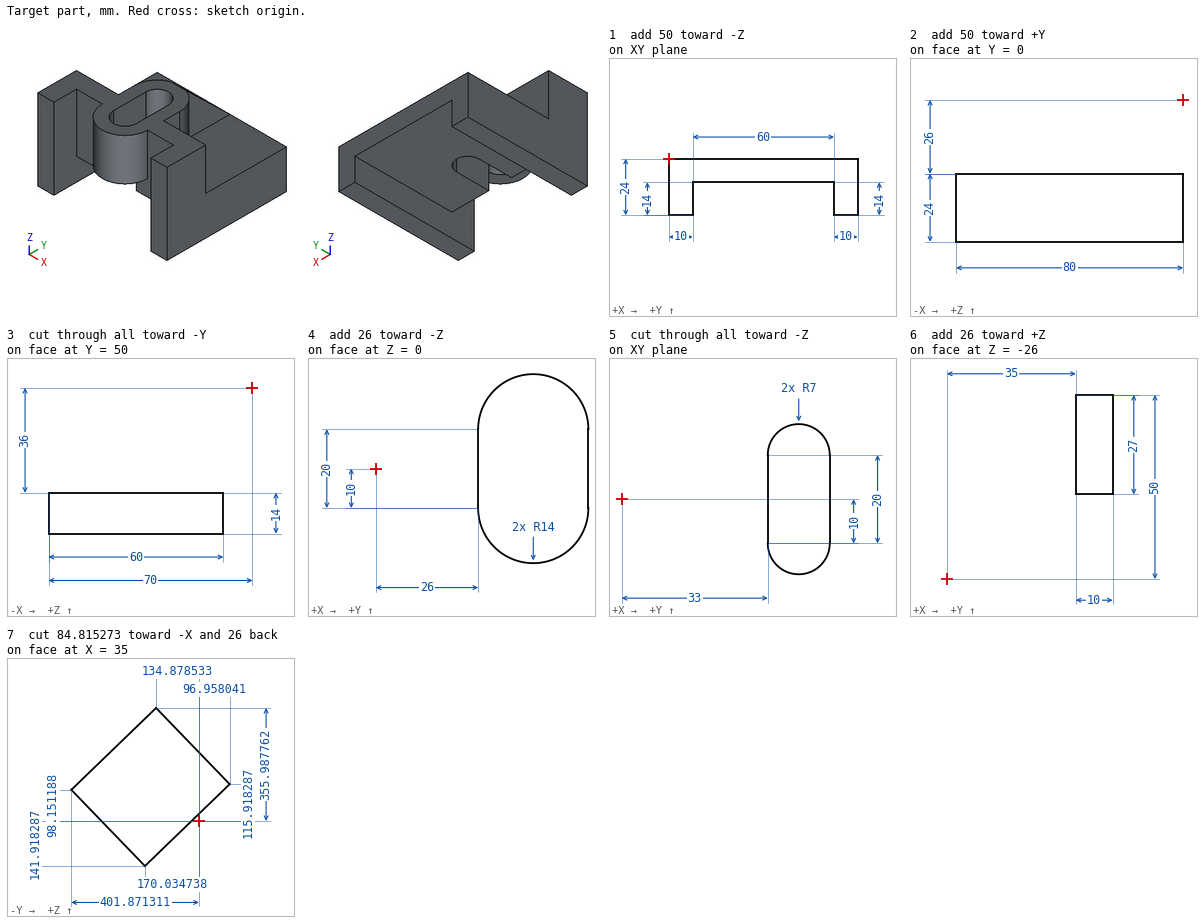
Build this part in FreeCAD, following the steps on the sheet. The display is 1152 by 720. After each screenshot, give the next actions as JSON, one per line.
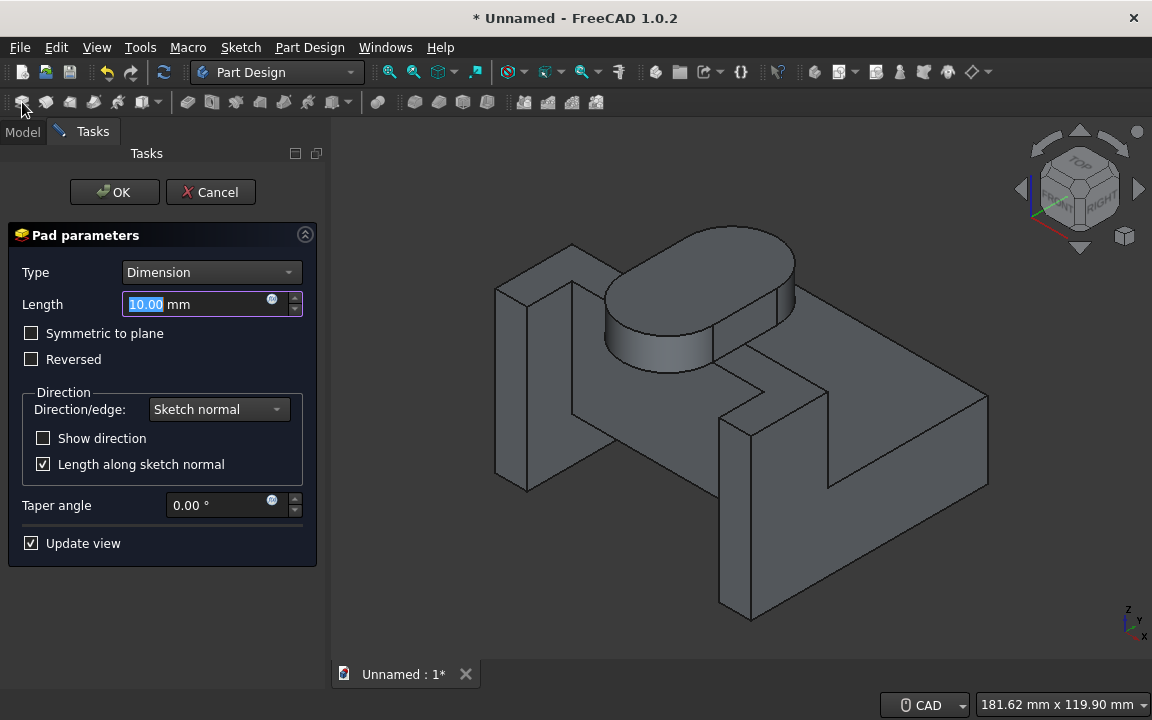
{"action": "type", "text": "26"}
{"action": "key", "text": "Tab"}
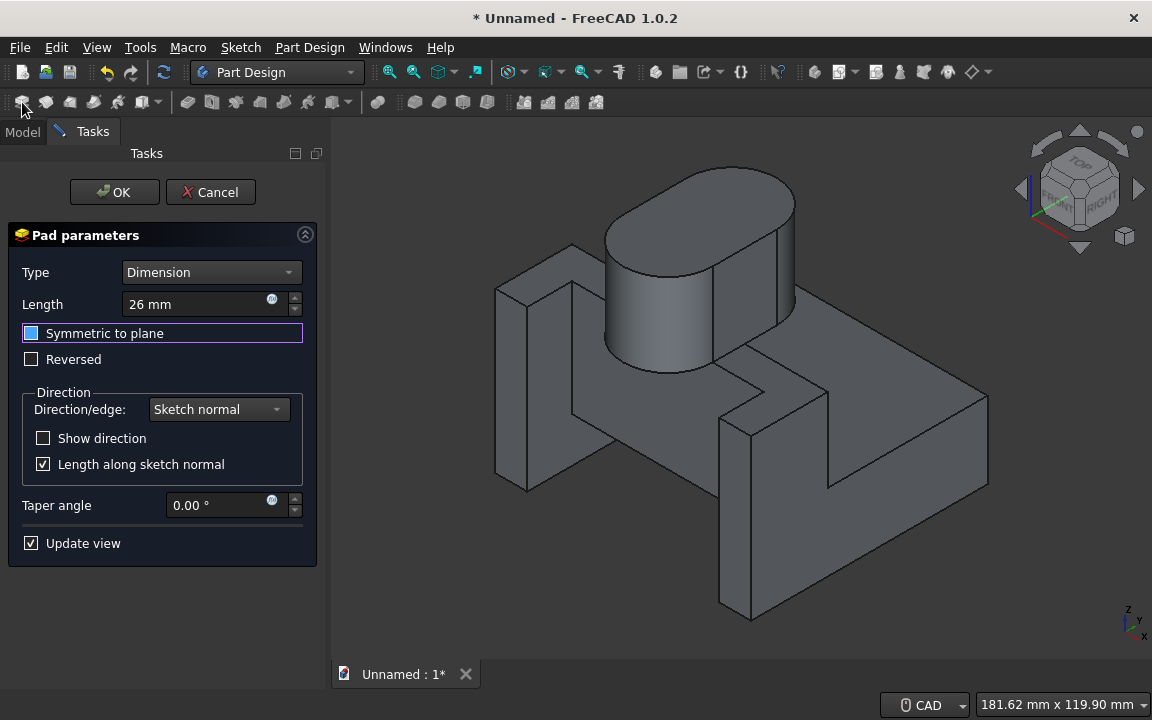
{"action": "left_click", "coordinate": [30, 359]}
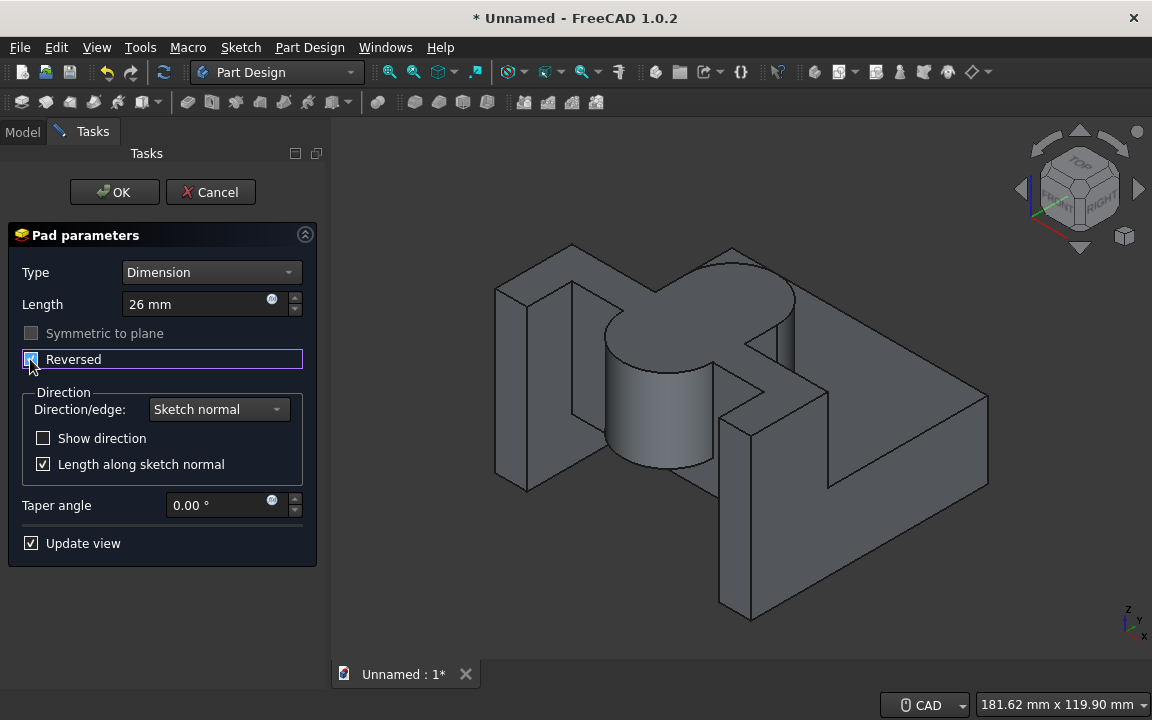
{"action": "left_click", "coordinate": [115, 192]}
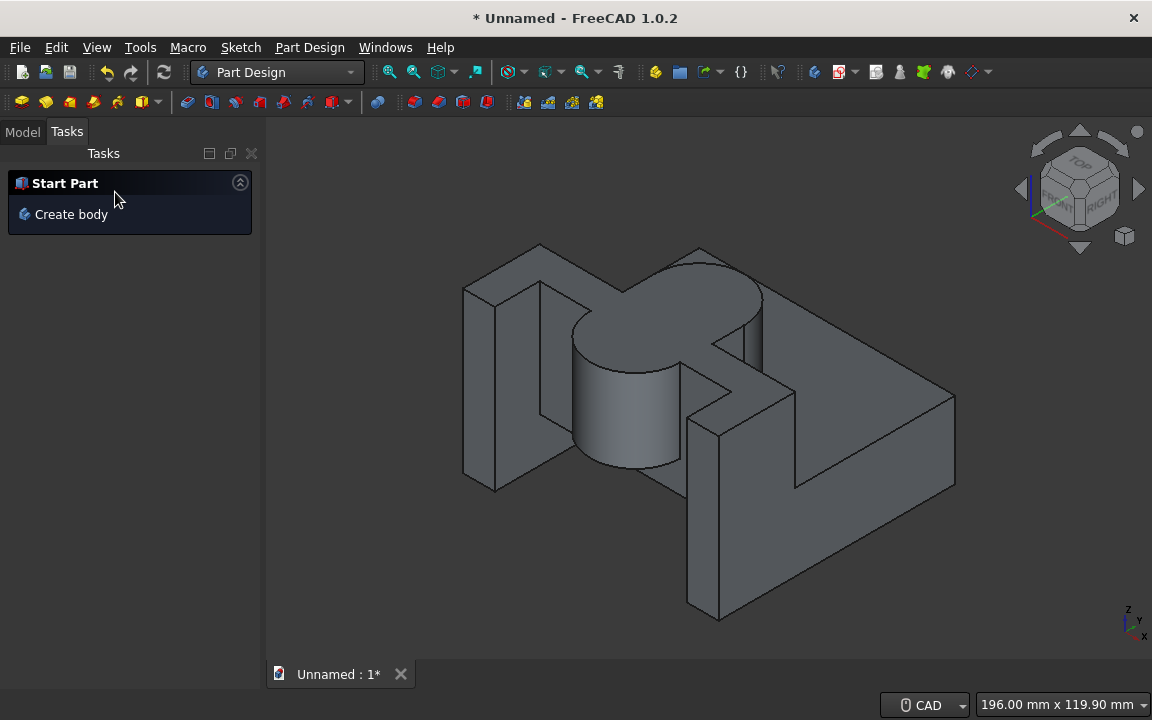
{"action": "left_click", "coordinate": [840, 72]}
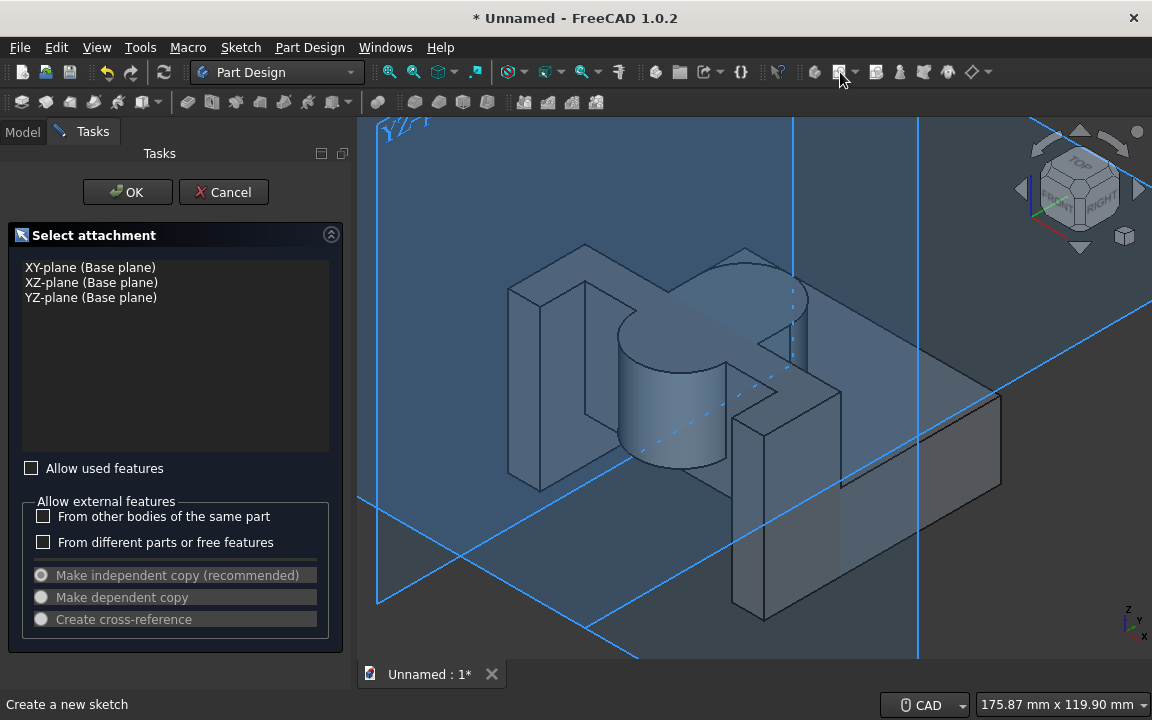
{"action": "left_click", "coordinate": [82, 268]}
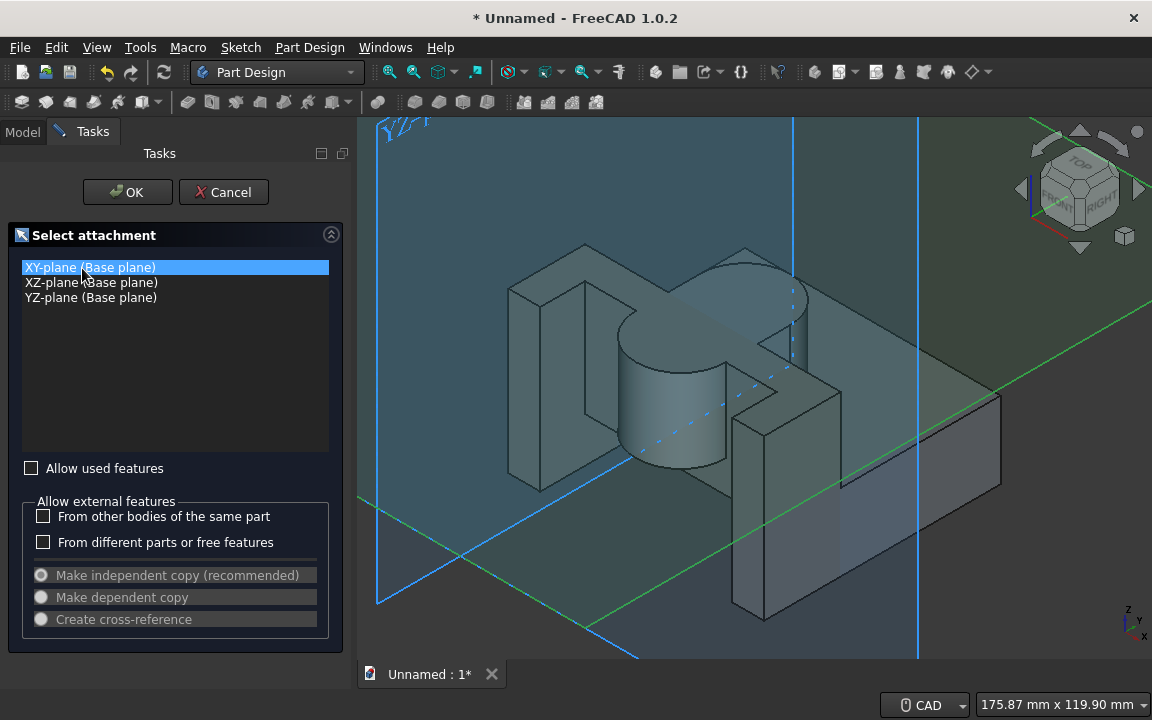
{"action": "left_click", "coordinate": [128, 192]}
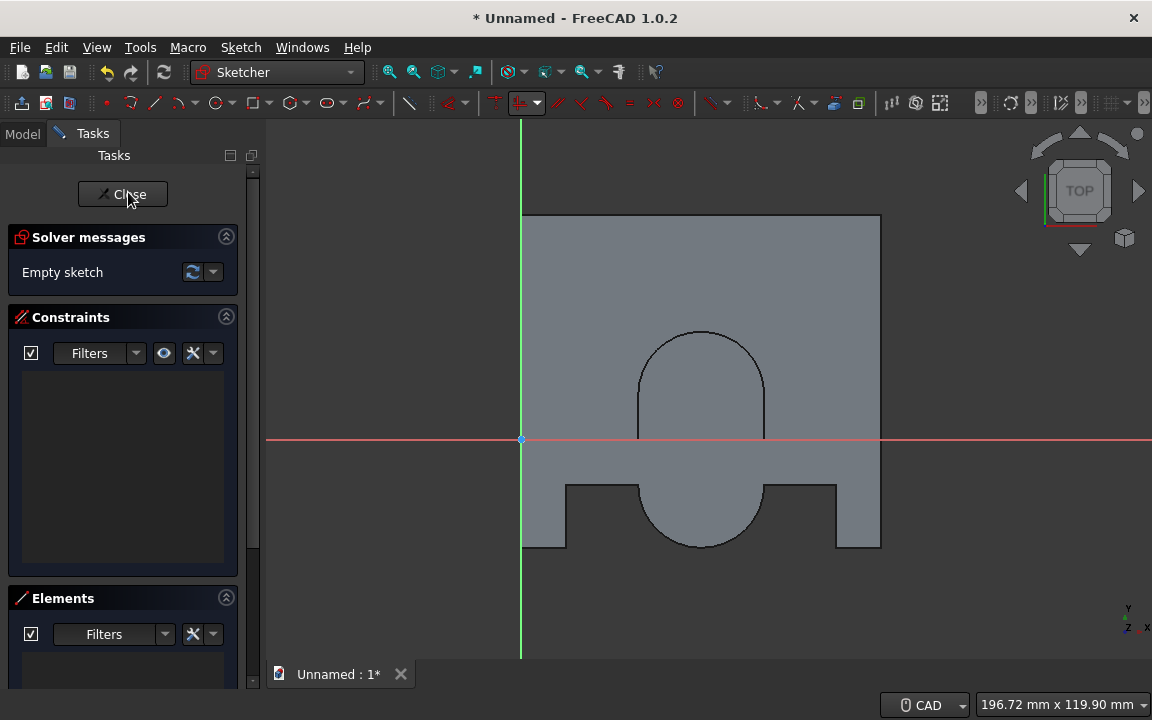
{"action": "scroll", "coordinate": [616, 481], "scroll_direction": "up", "scroll_amount": 4}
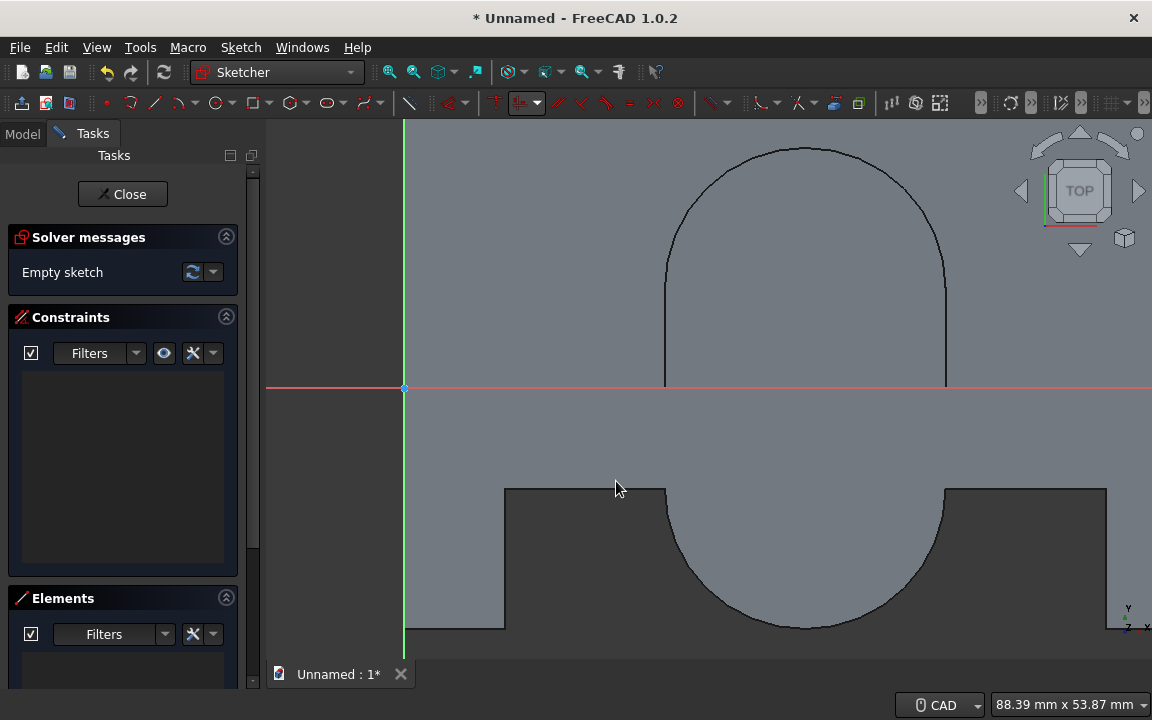
{"action": "key", "text": "g s"}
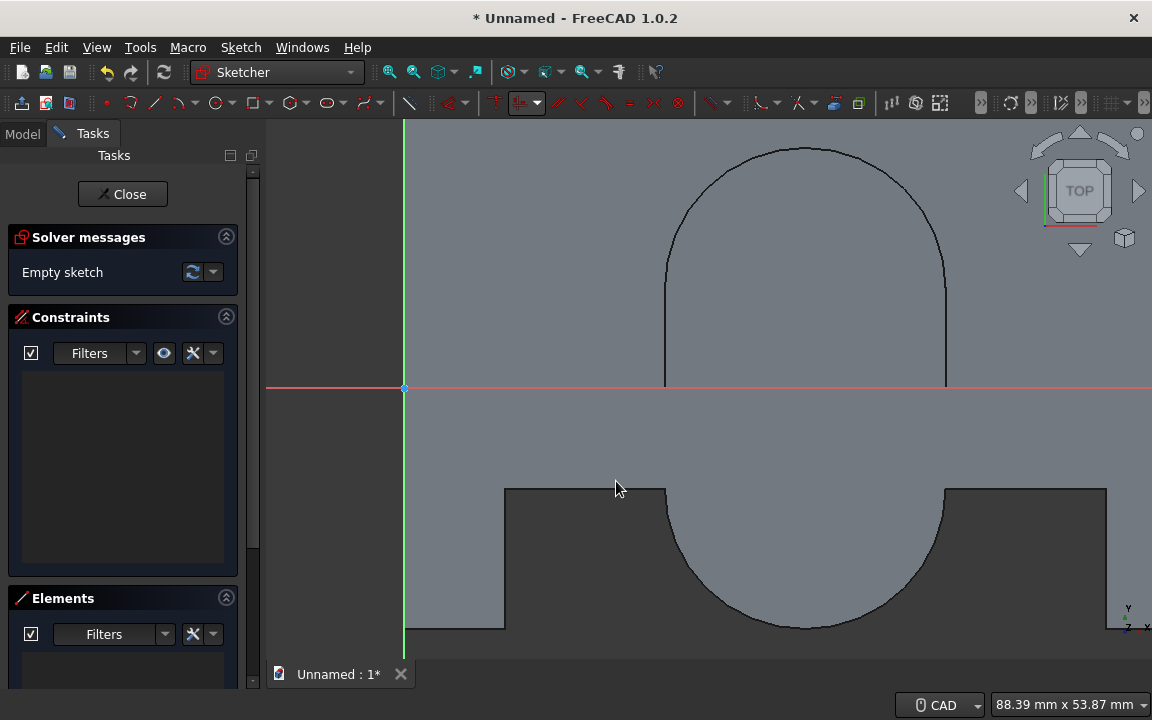
{"action": "left_click", "coordinate": [805, 489]}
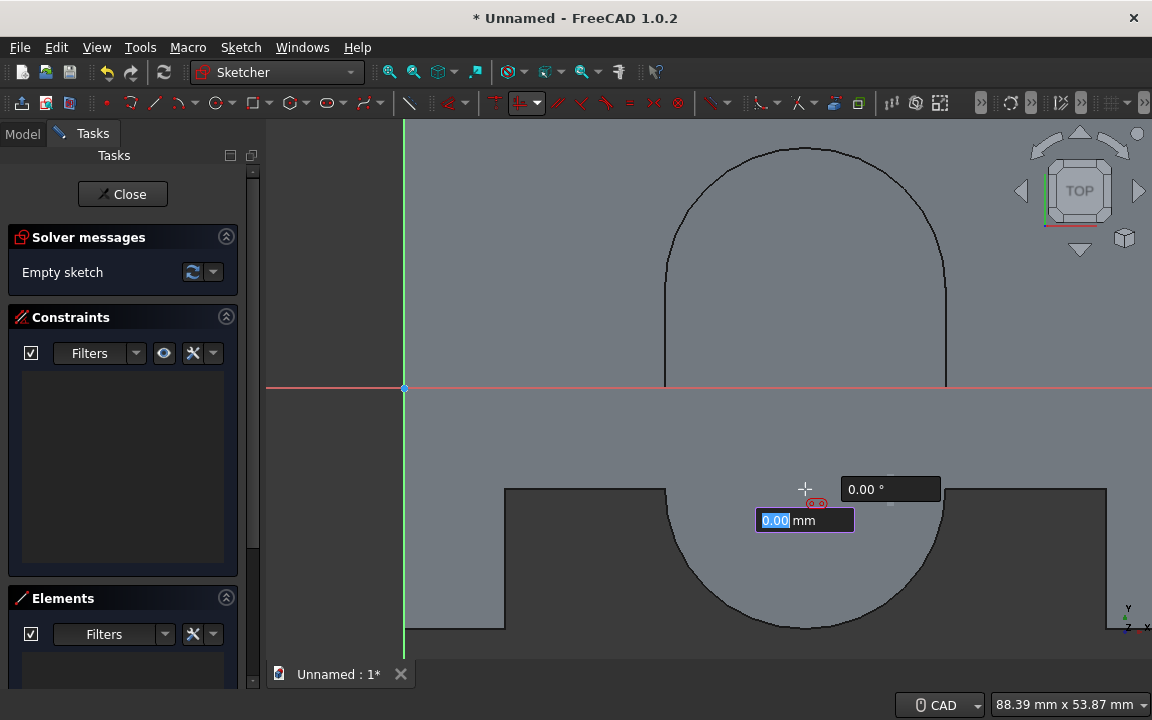
{"action": "left_click", "coordinate": [805, 288]}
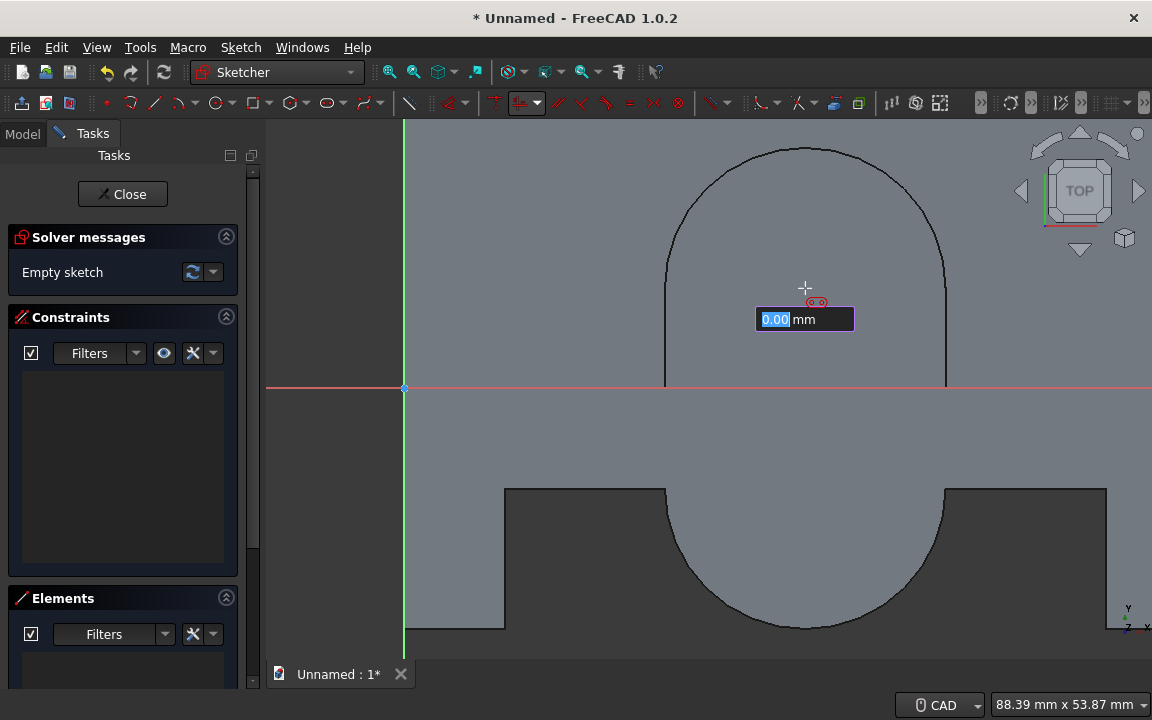
{"action": "left_click", "coordinate": [735, 358]}
{"action": "key", "text": "Escape"}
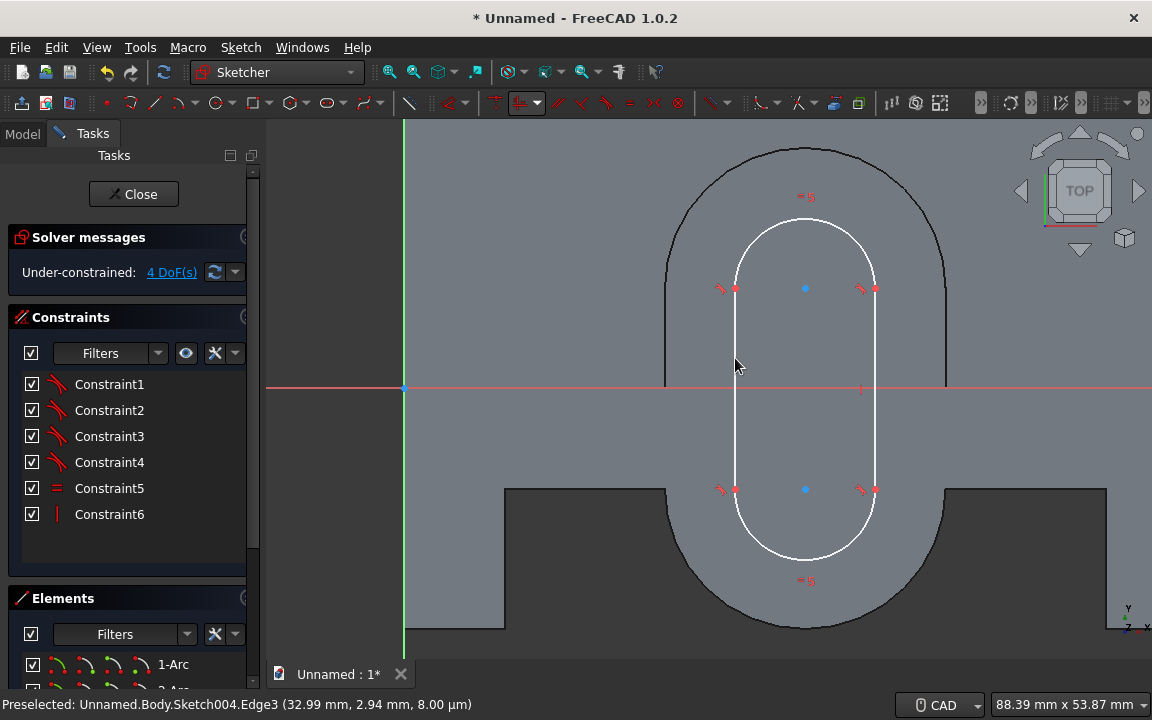
{"action": "key", "text": "d"}